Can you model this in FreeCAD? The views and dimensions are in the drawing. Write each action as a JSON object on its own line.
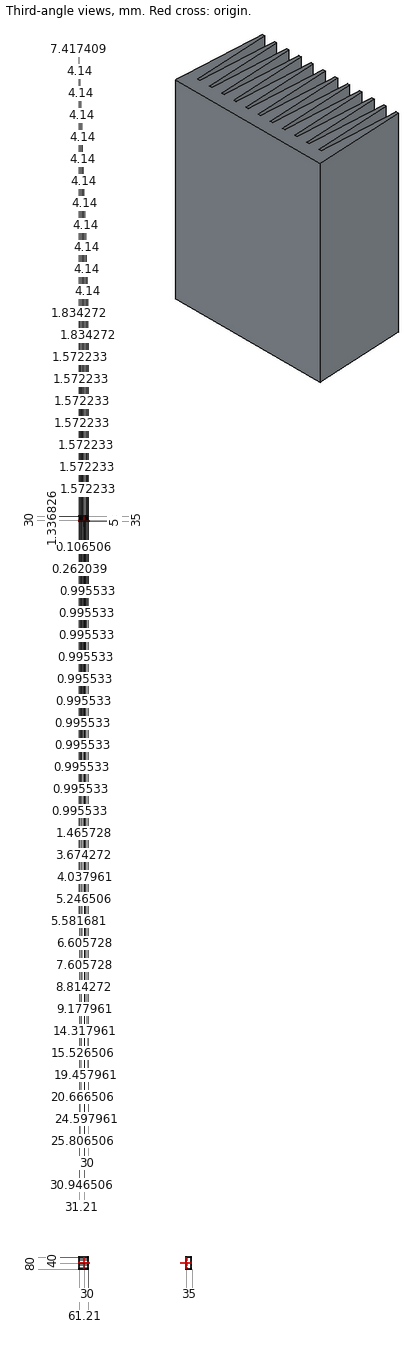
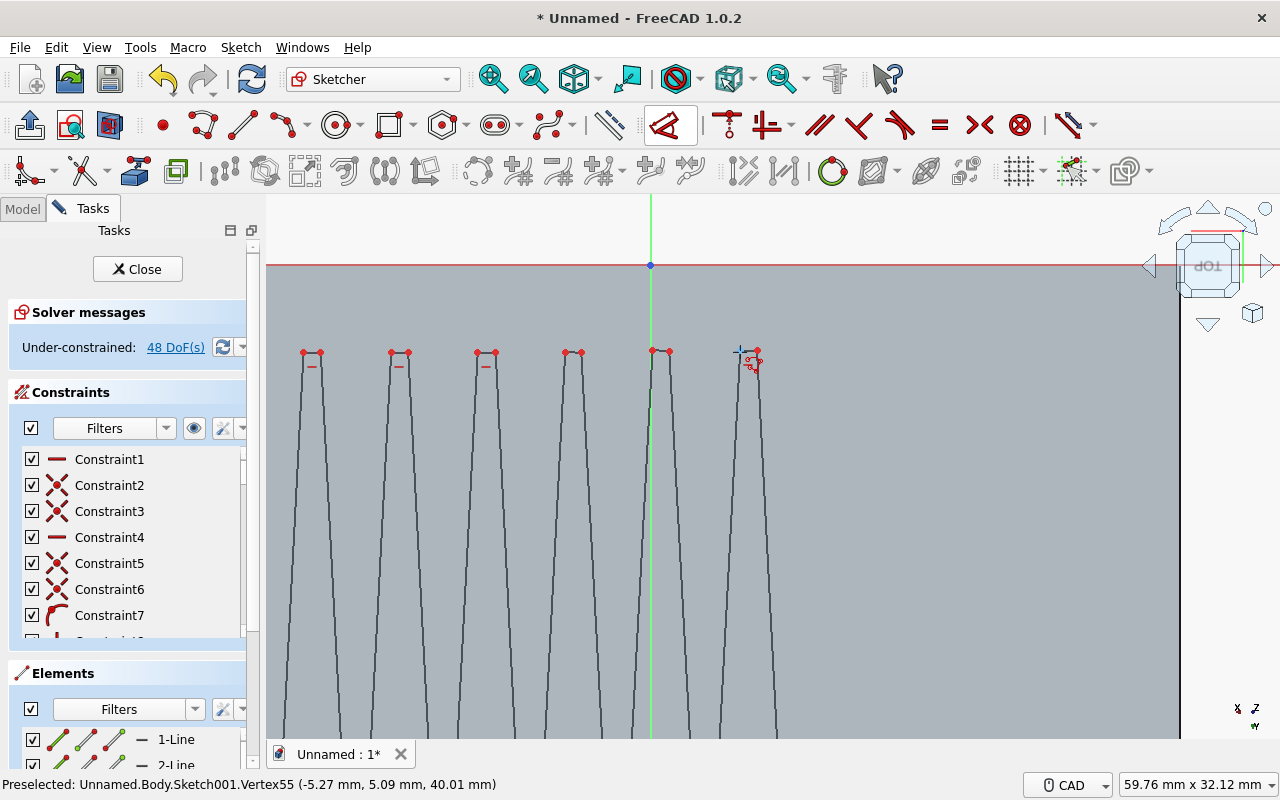
{"action": "left_click", "coordinate": [827, 350]}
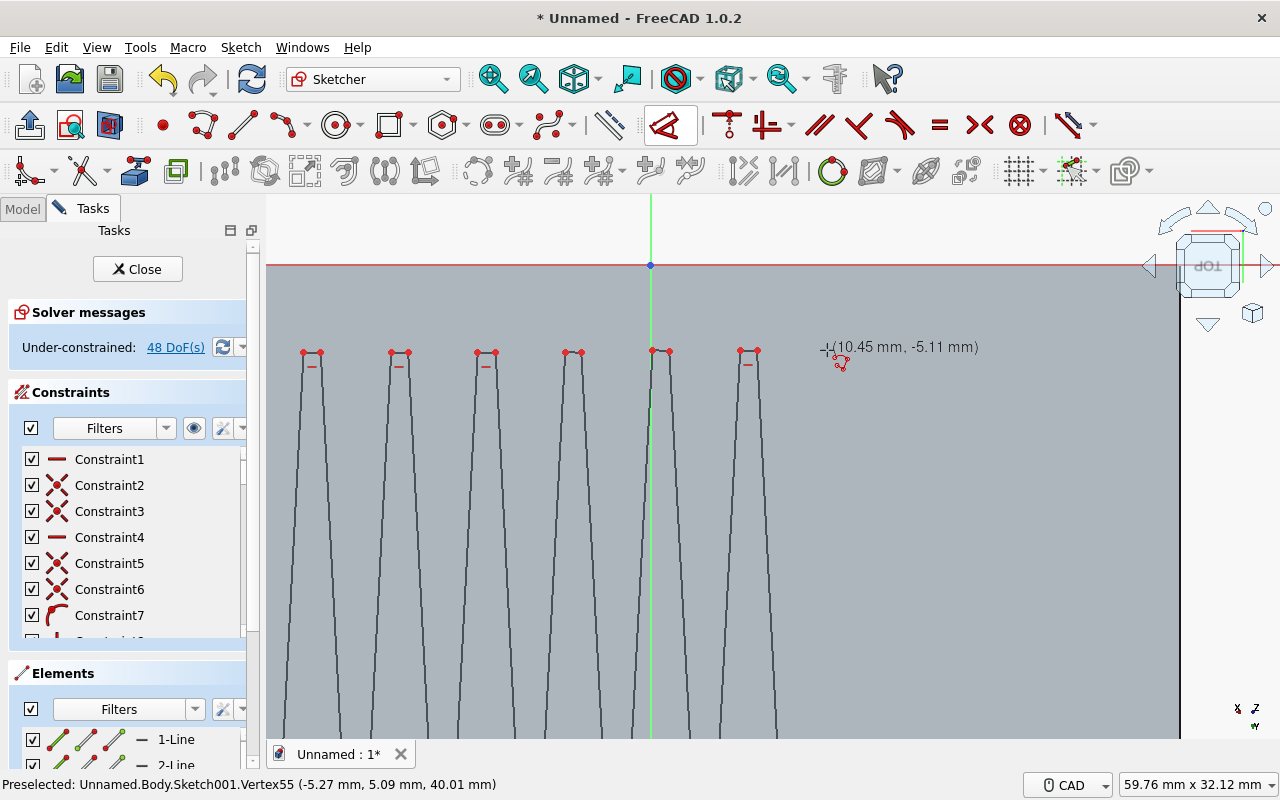
{"action": "scroll", "coordinate": [757, 350], "scroll_direction": "down", "scroll_amount": 3}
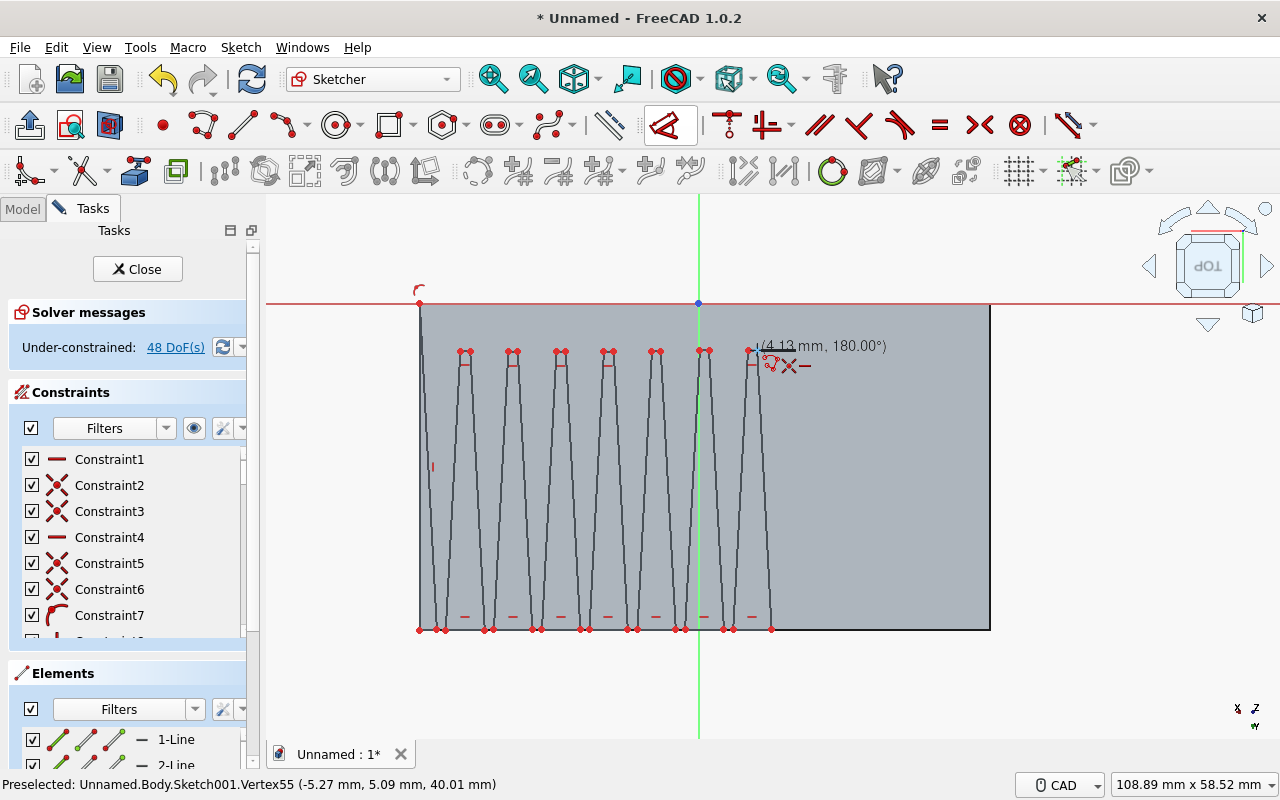
{"action": "scroll", "coordinate": [781, 630], "scroll_direction": "up", "scroll_amount": 3}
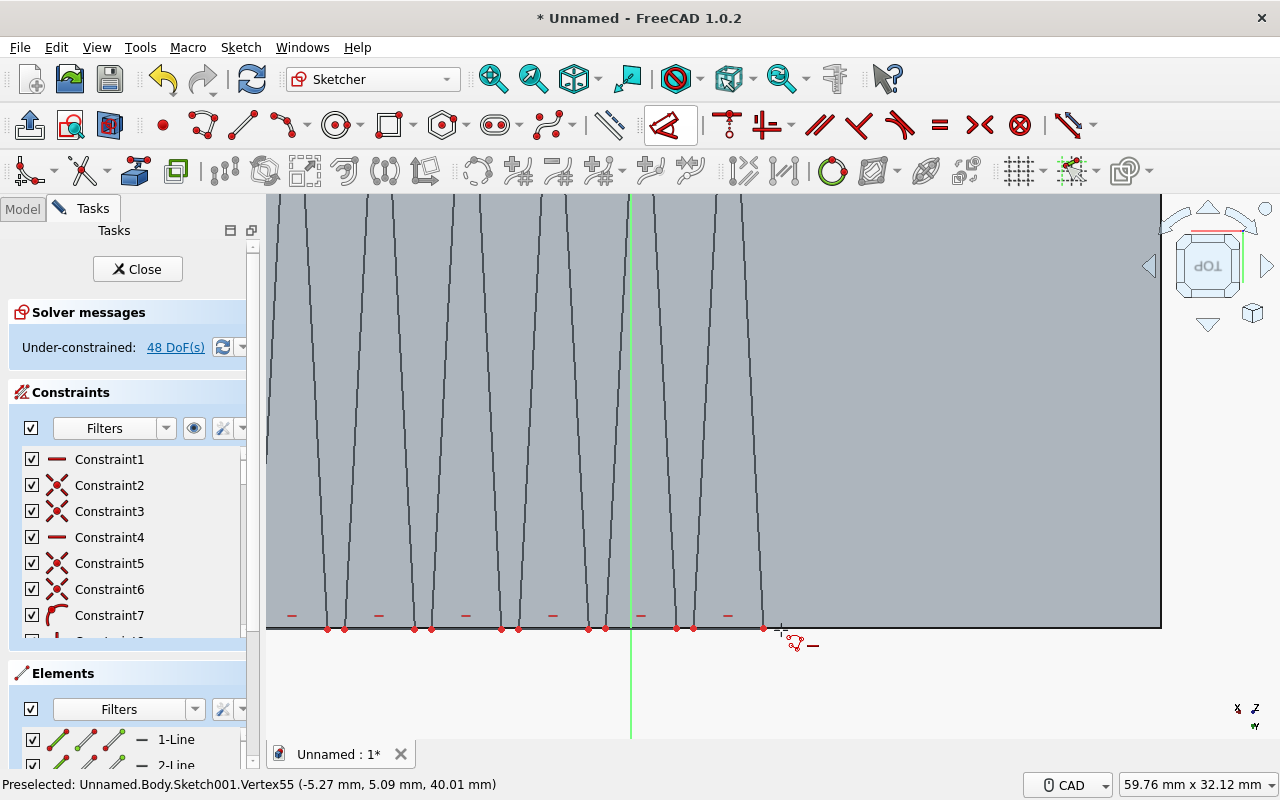
{"action": "left_click", "coordinate": [781, 628]}
{"action": "left_click", "coordinate": [851, 628]}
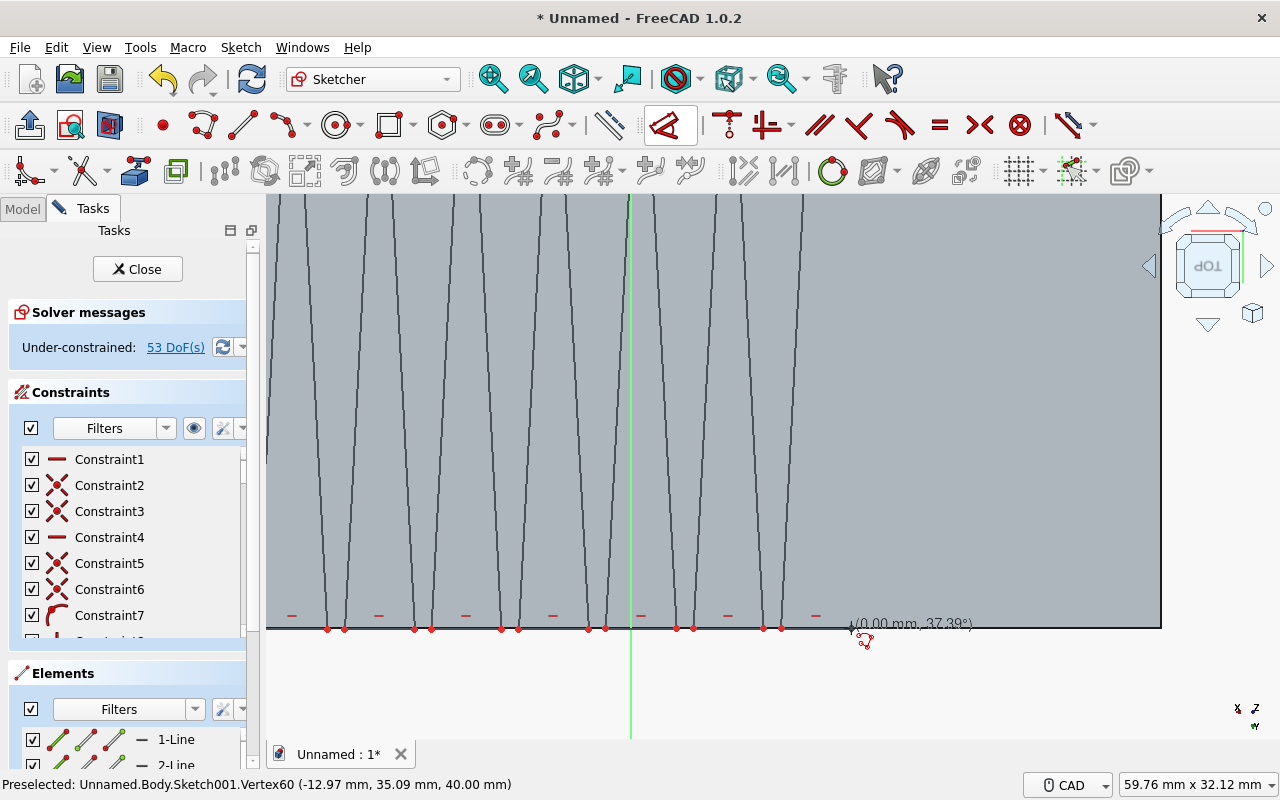
{"action": "scroll", "coordinate": [781, 631], "scroll_direction": "down", "scroll_amount": 3}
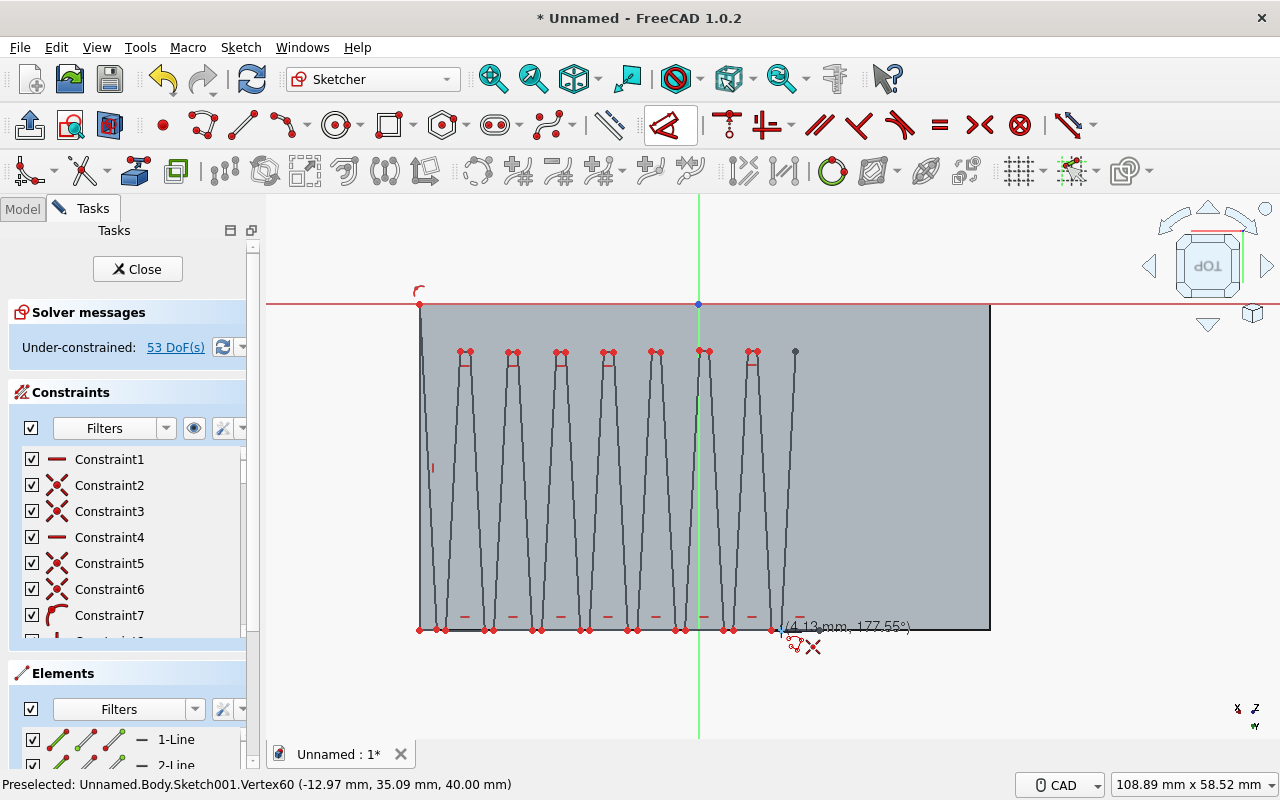
{"action": "scroll", "coordinate": [805, 351], "scroll_direction": "up", "scroll_amount": 3}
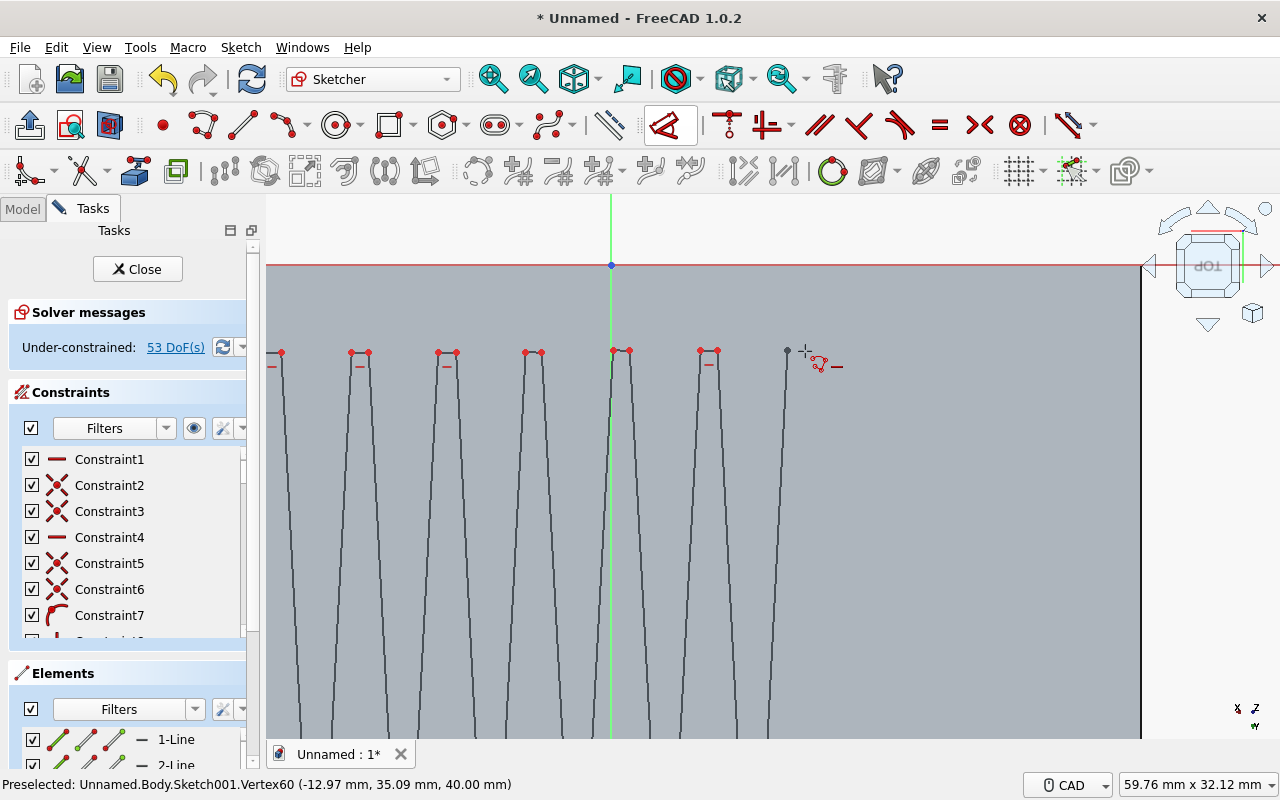
{"action": "left_click", "coordinate": [804, 350]}
{"action": "left_click", "coordinate": [787, 351]}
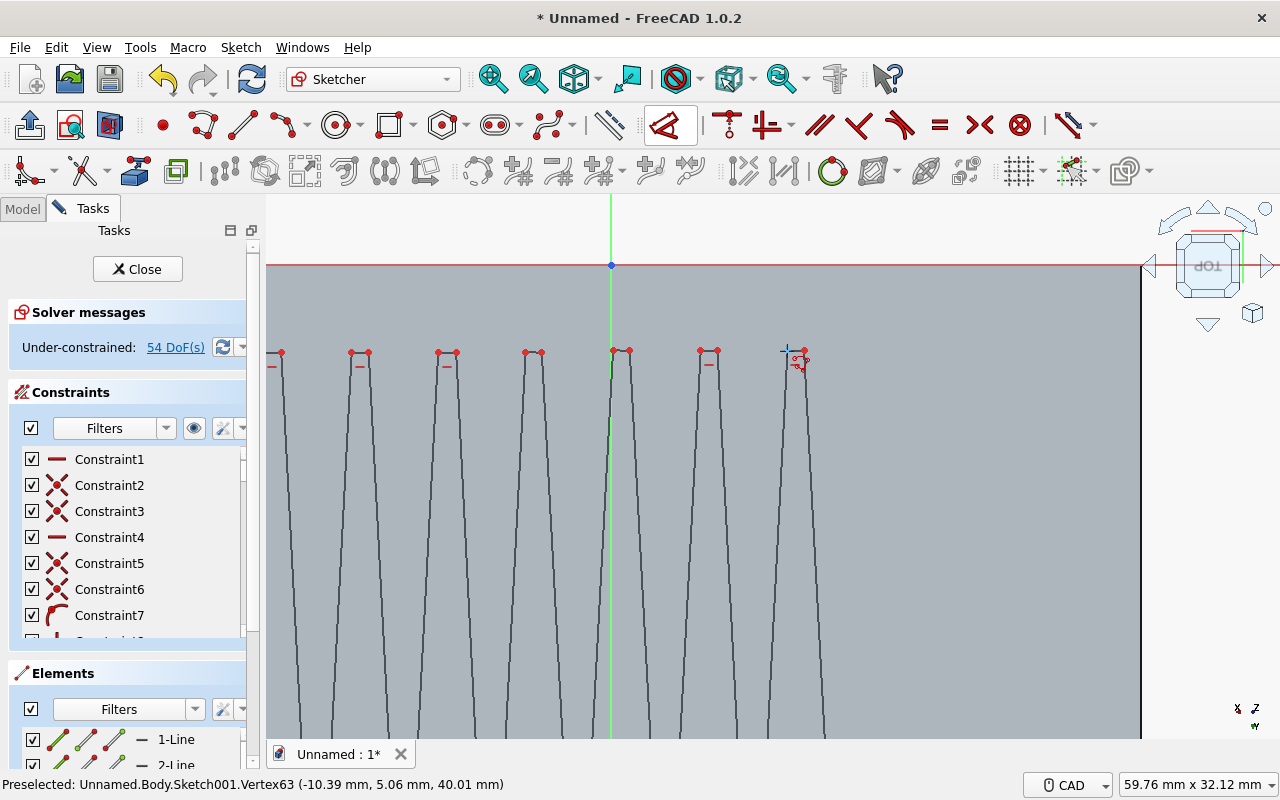
{"action": "left_click", "coordinate": [875, 350]}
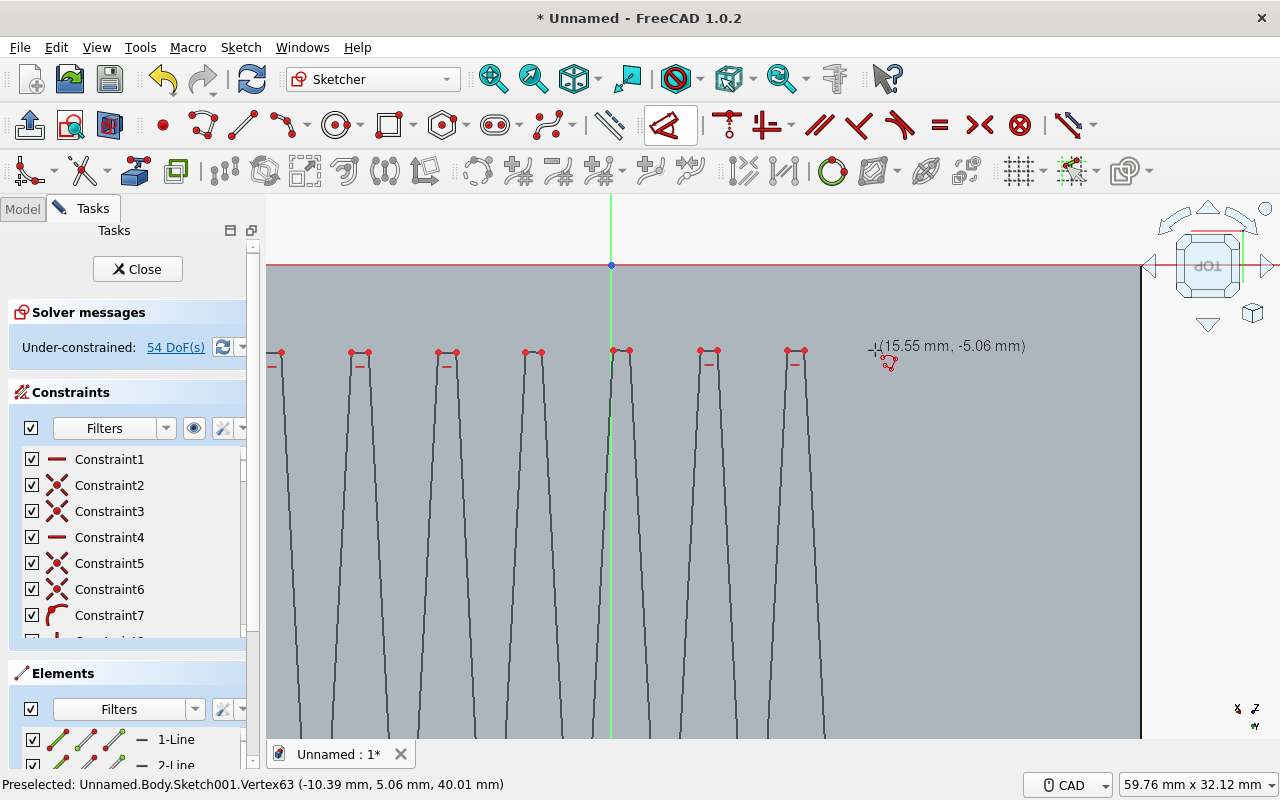
{"action": "scroll", "coordinate": [805, 350], "scroll_direction": "down", "scroll_amount": 3}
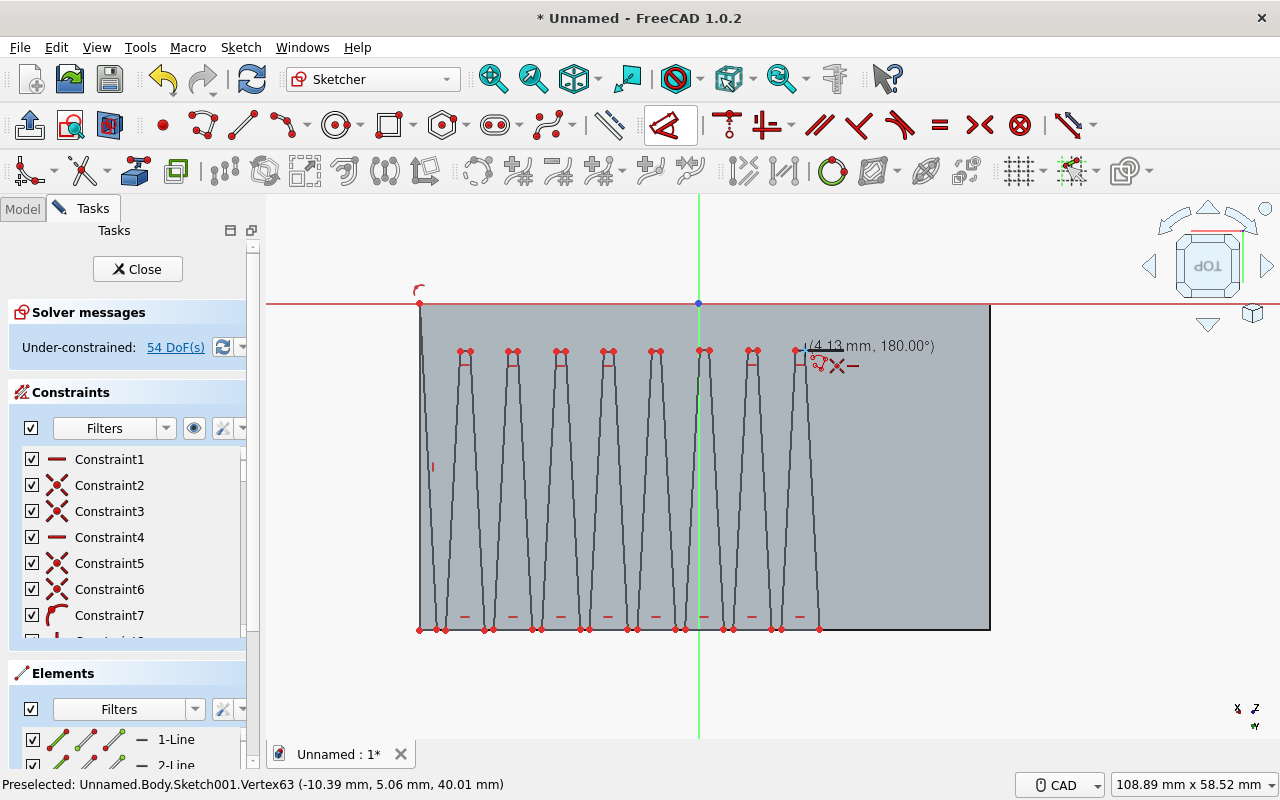
{"action": "scroll", "coordinate": [829, 630], "scroll_direction": "up", "scroll_amount": 3}